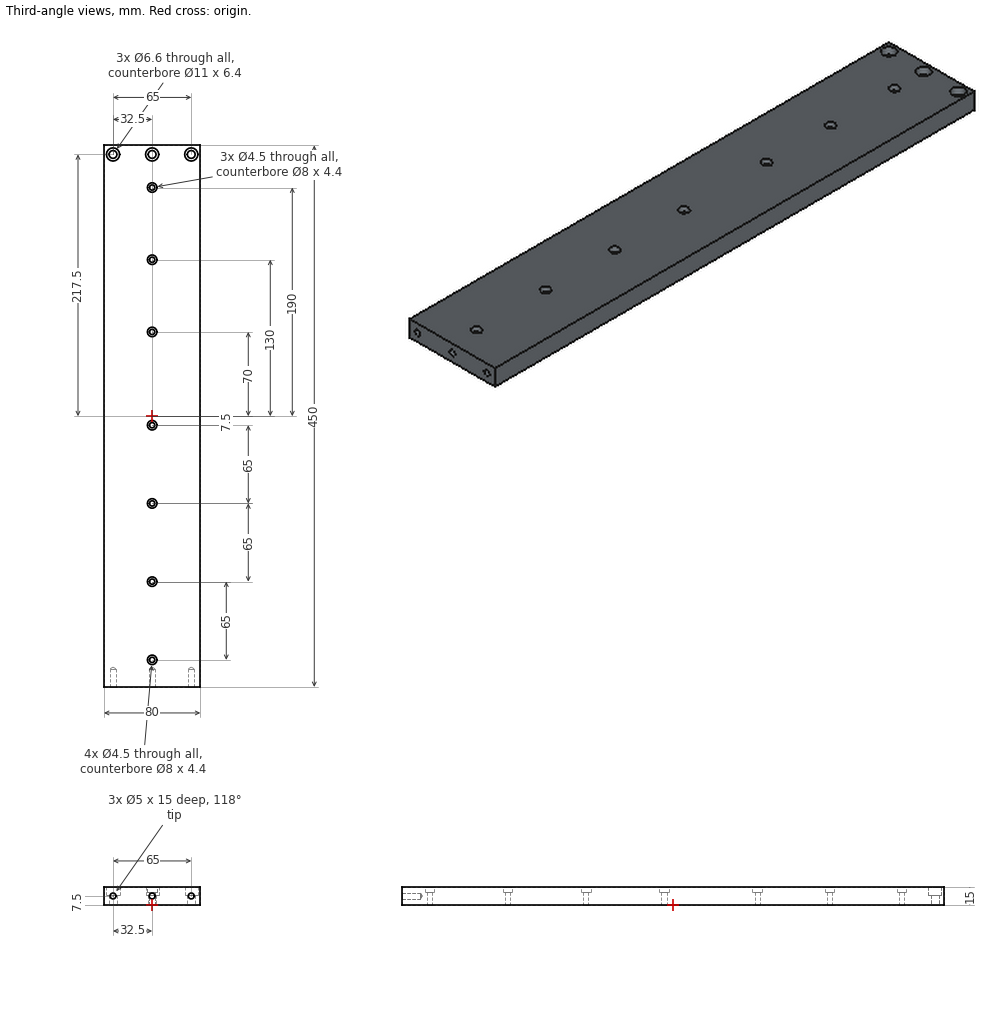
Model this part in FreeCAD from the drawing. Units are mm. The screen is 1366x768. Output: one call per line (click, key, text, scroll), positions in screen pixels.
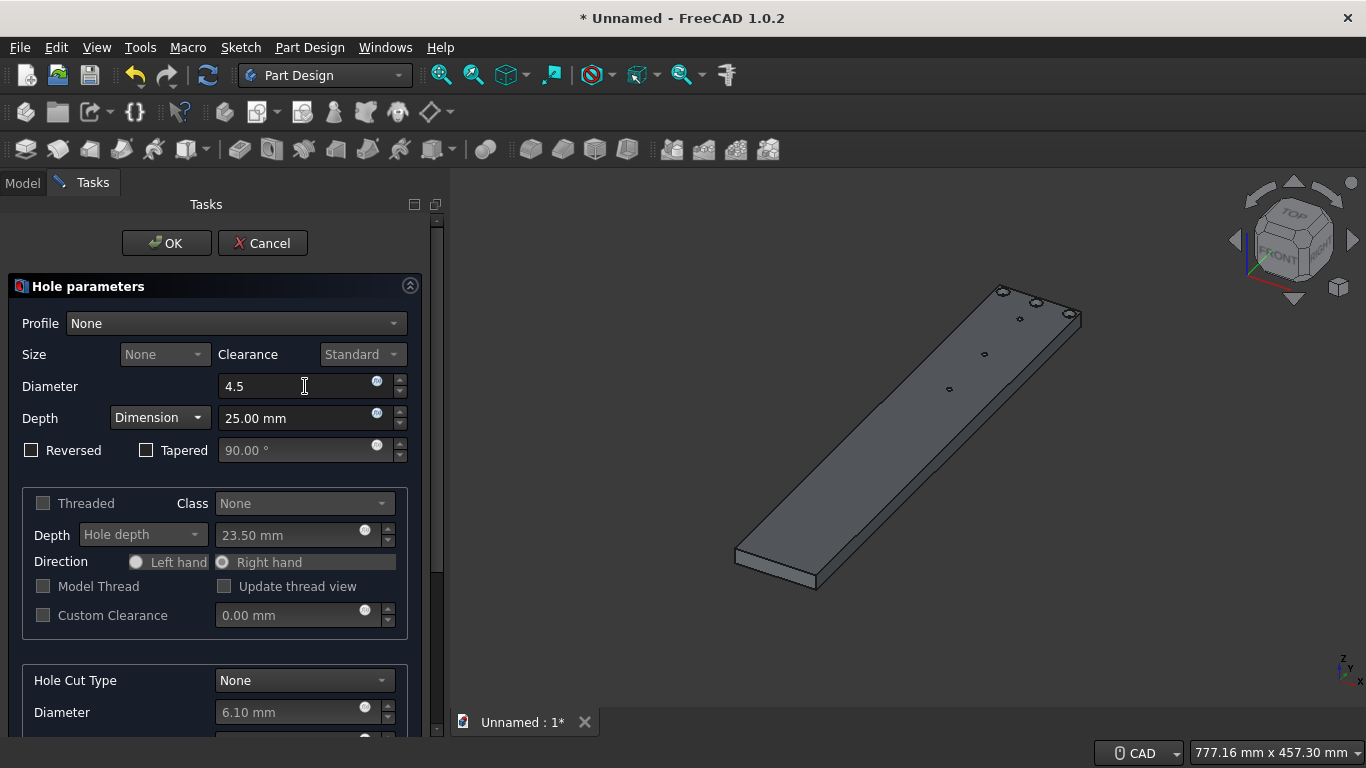
click(161, 418)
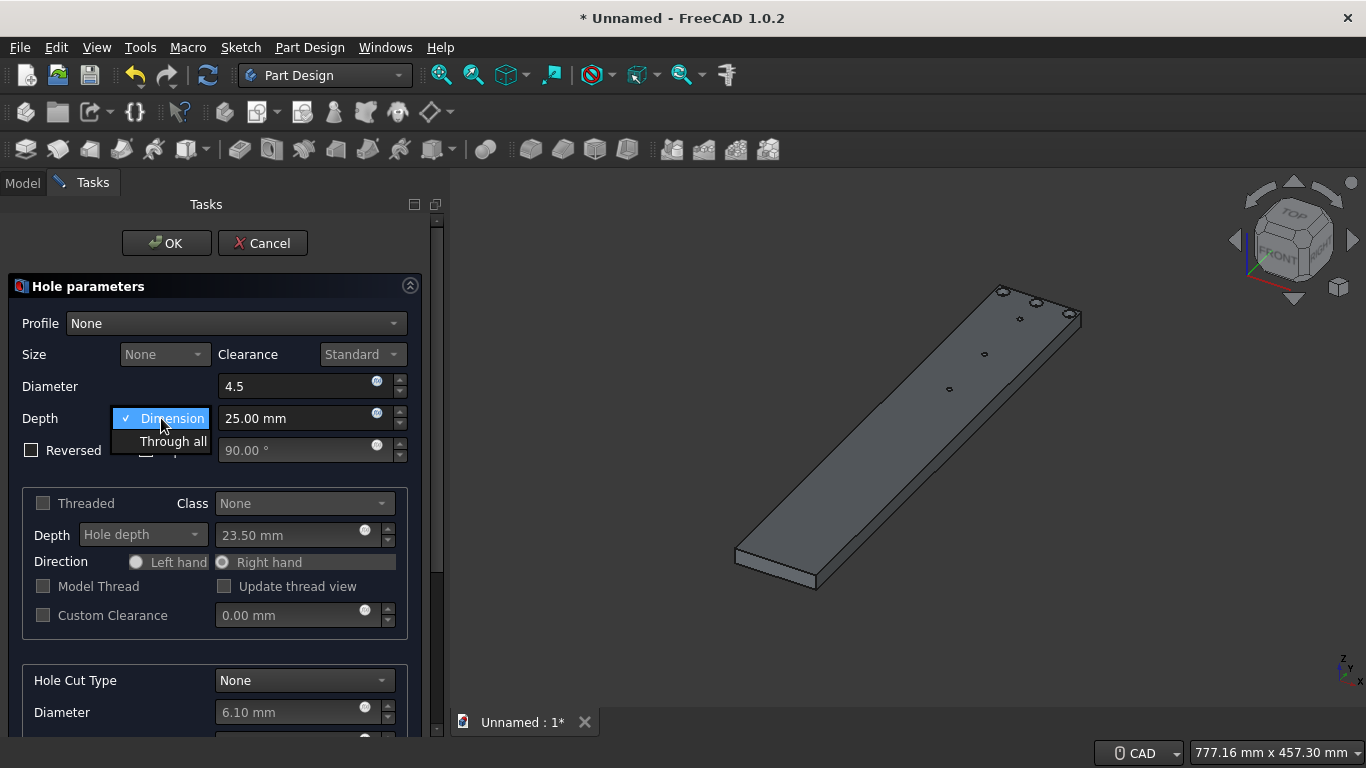
click(160, 442)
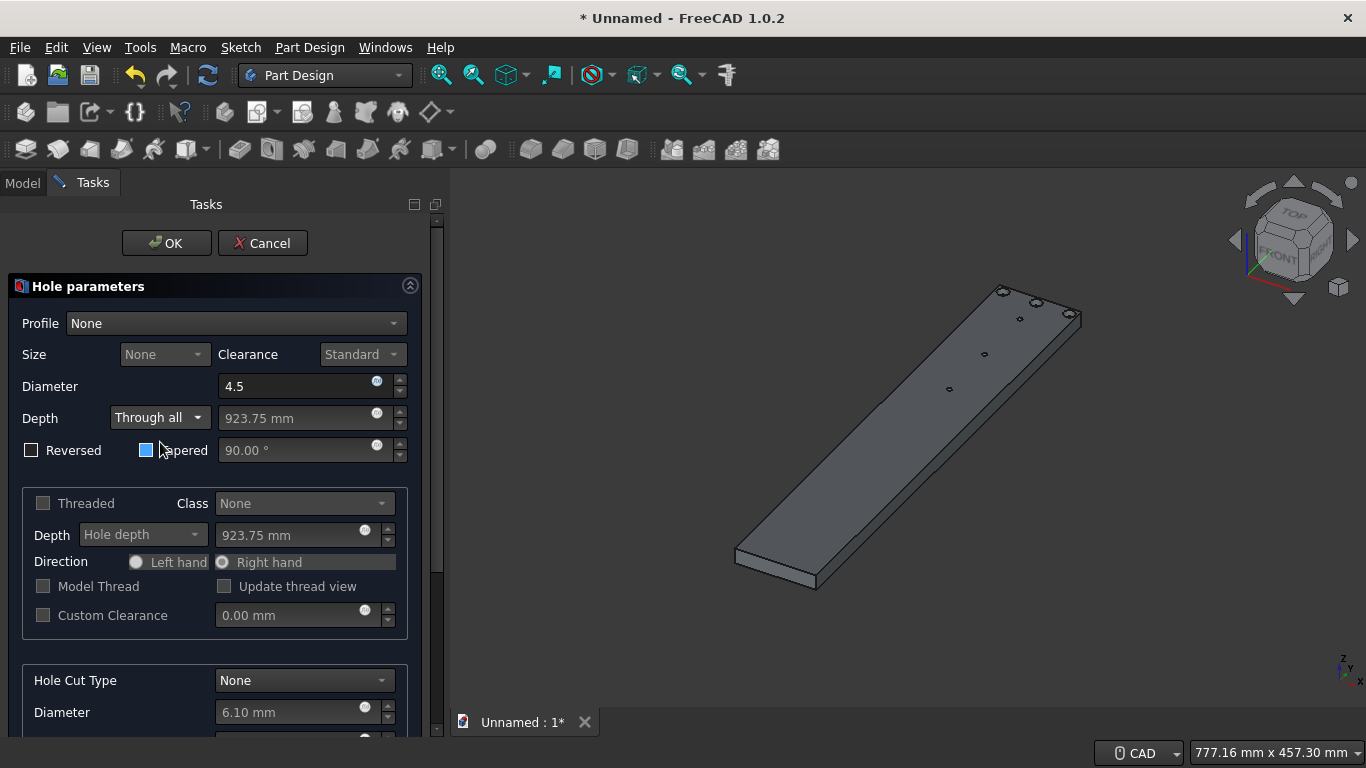
click(306, 680)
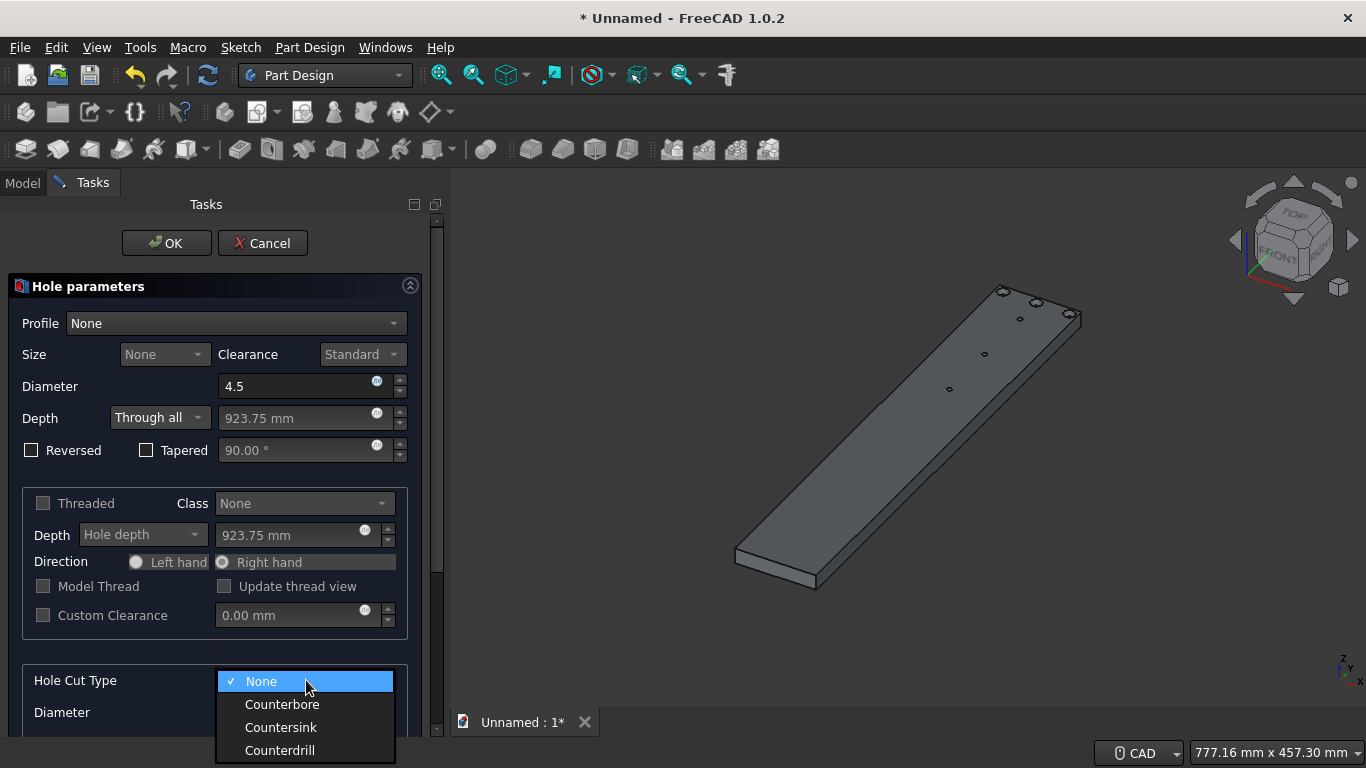
click(304, 704)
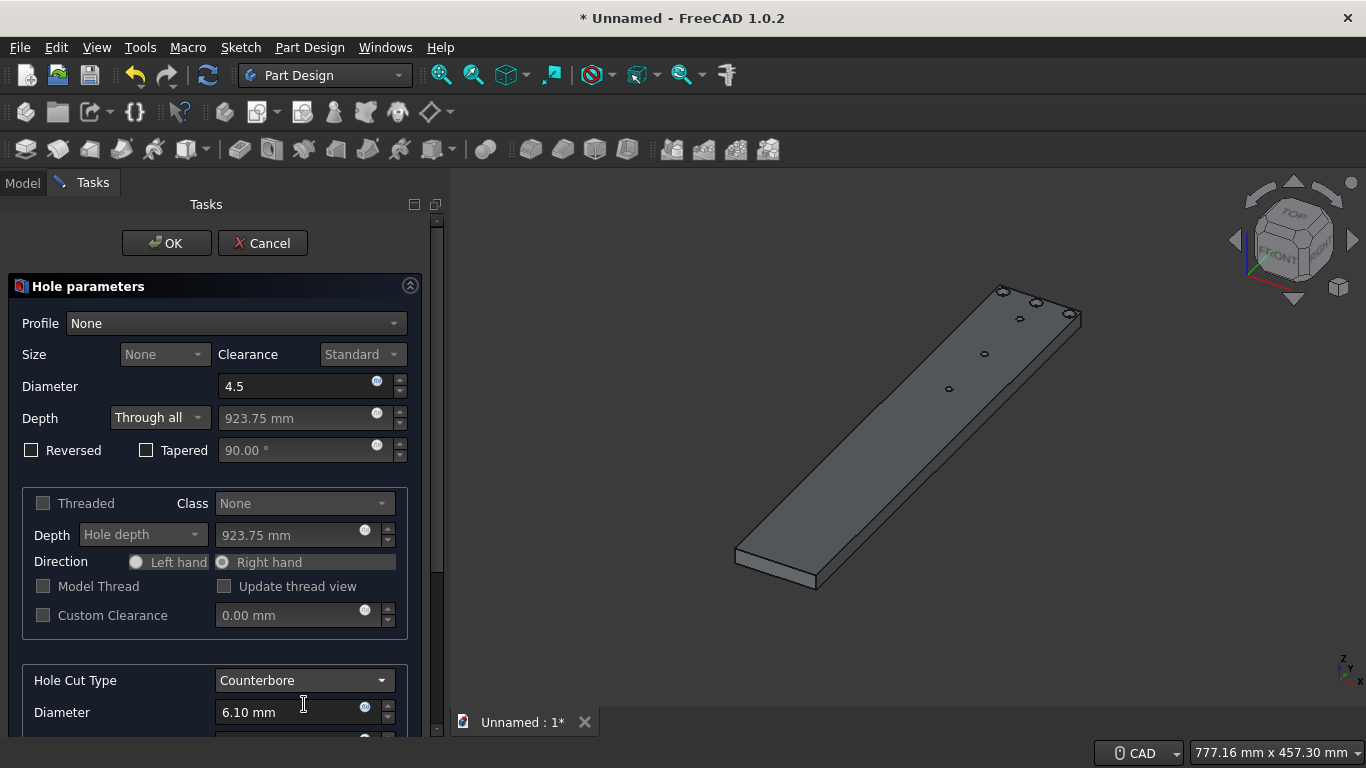
triple_click(298, 712)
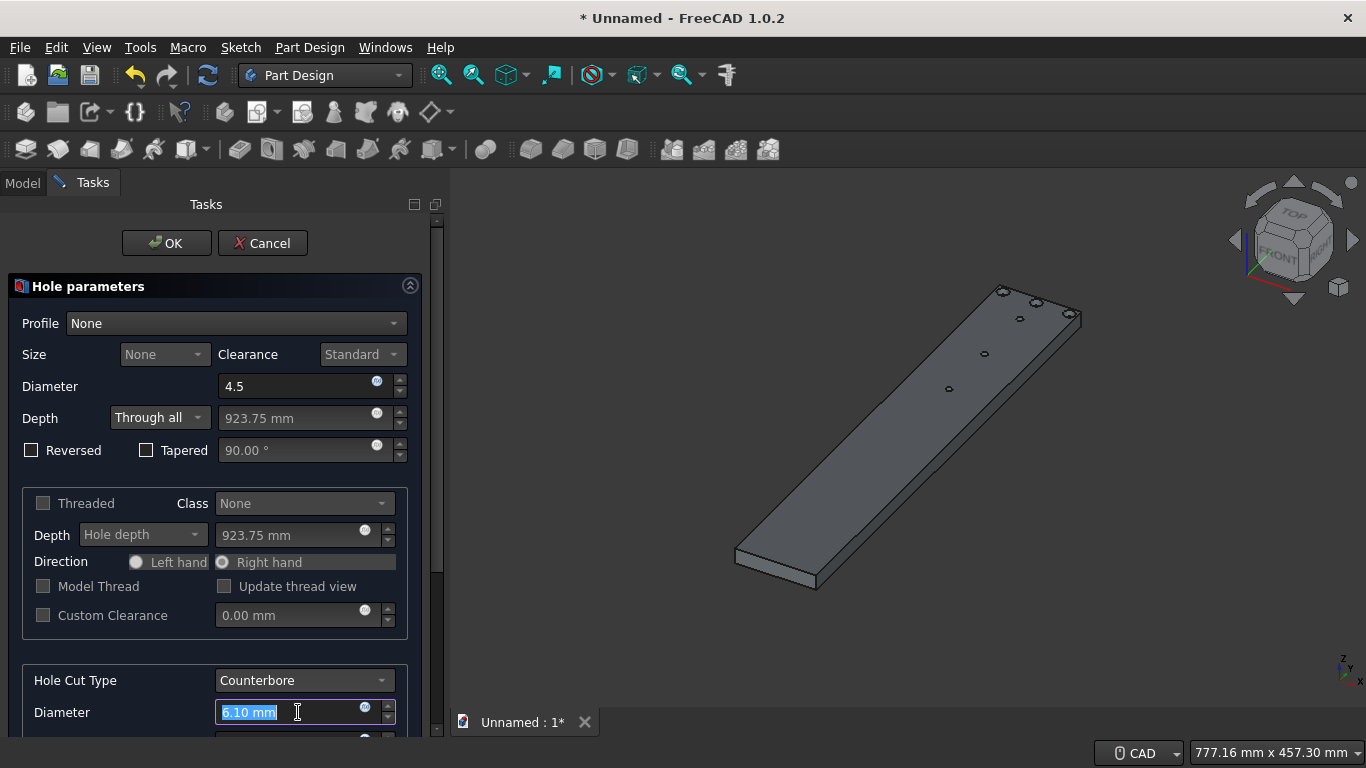
text(8)
key(Tab)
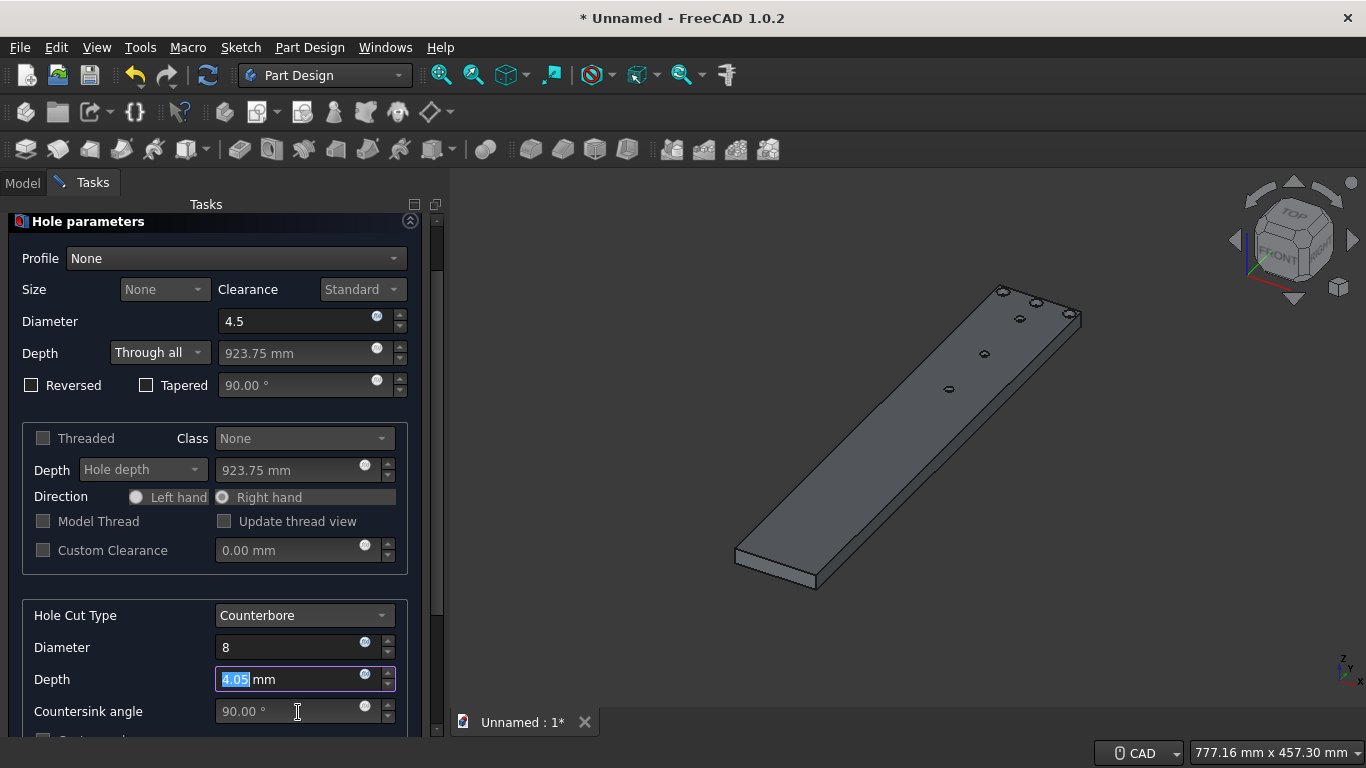
text(4.4)
key(Tab)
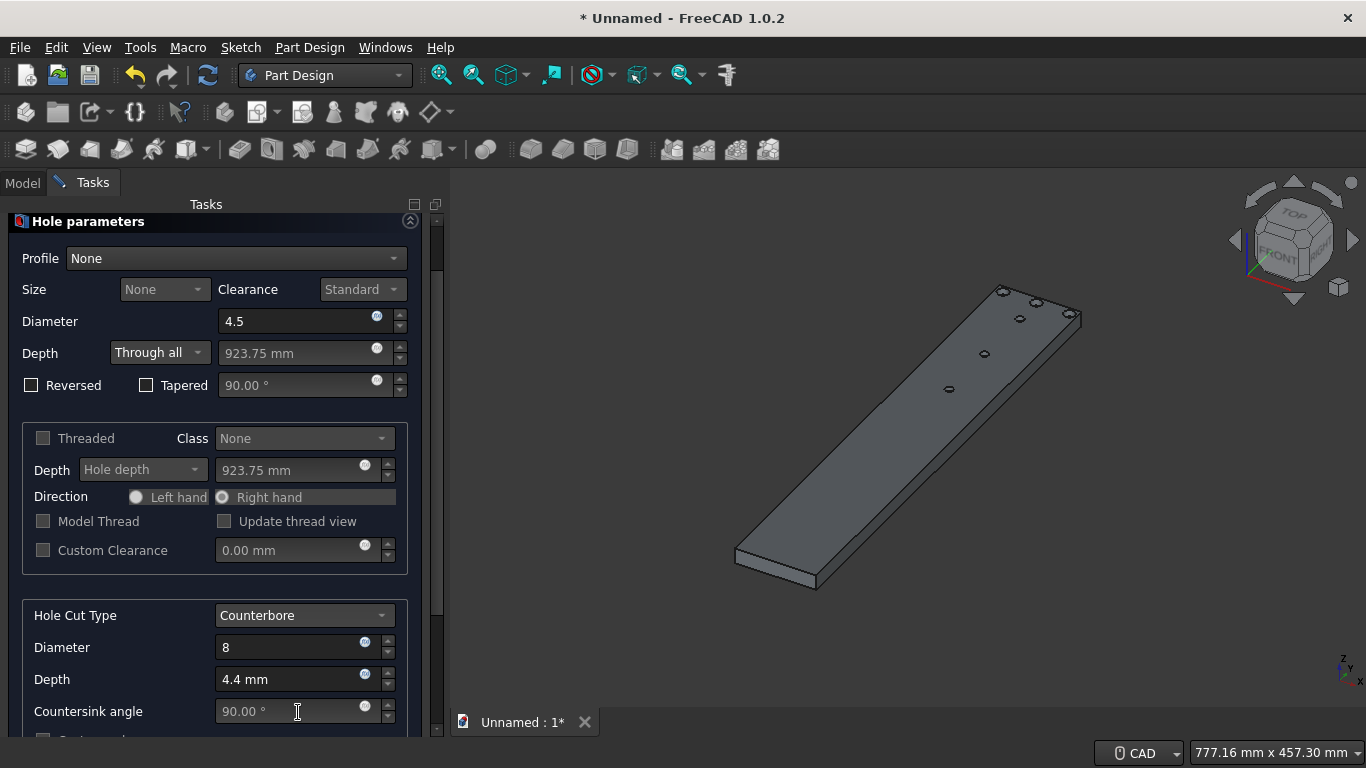
scroll(437, 475, up, 2)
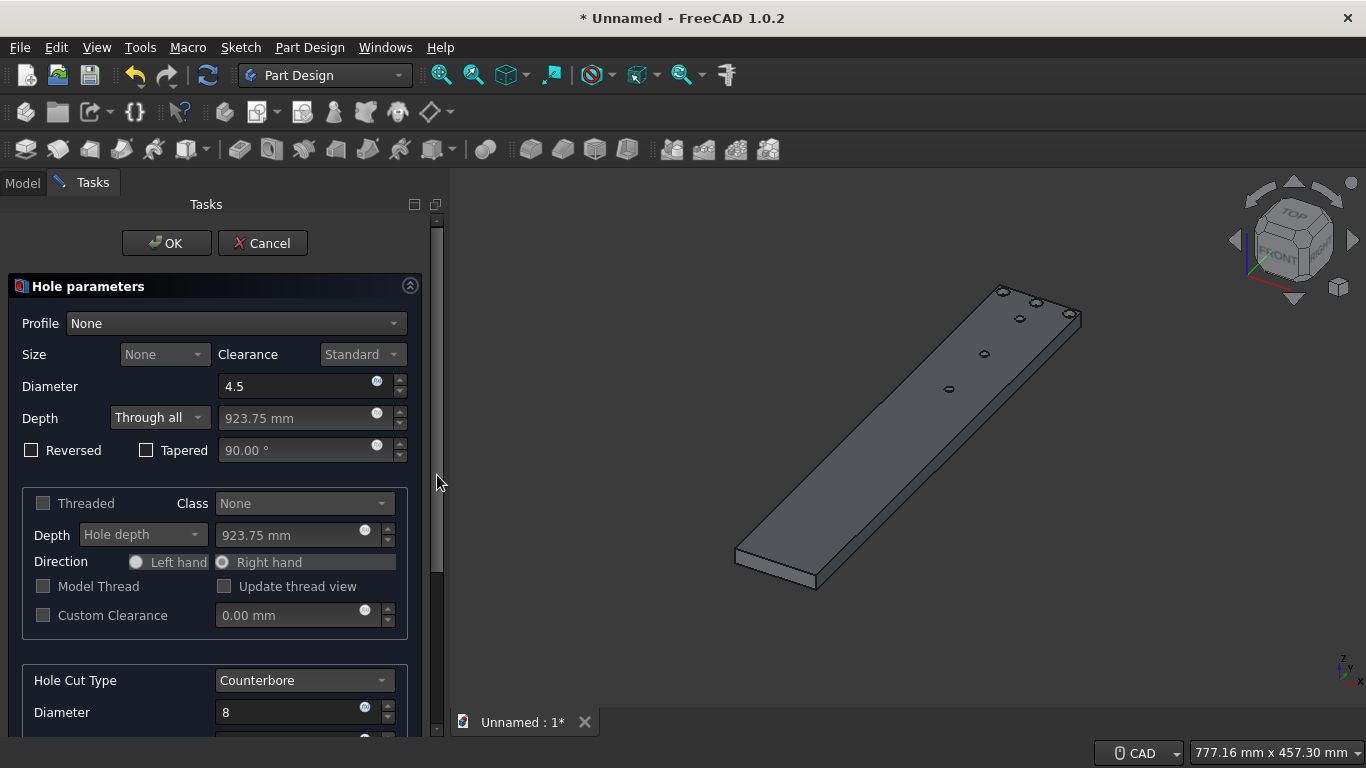
click(167, 243)